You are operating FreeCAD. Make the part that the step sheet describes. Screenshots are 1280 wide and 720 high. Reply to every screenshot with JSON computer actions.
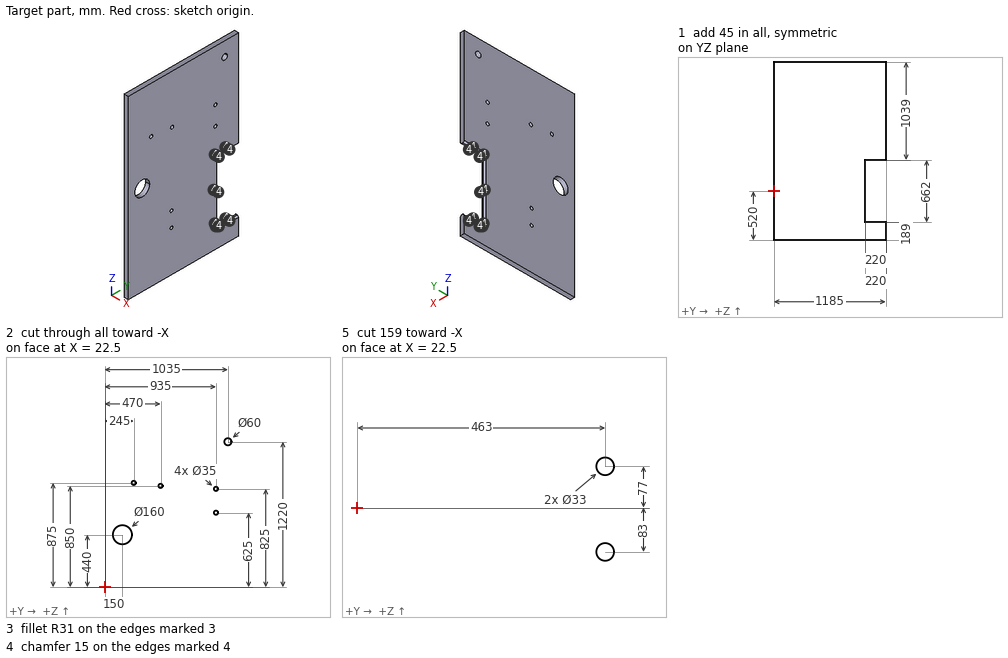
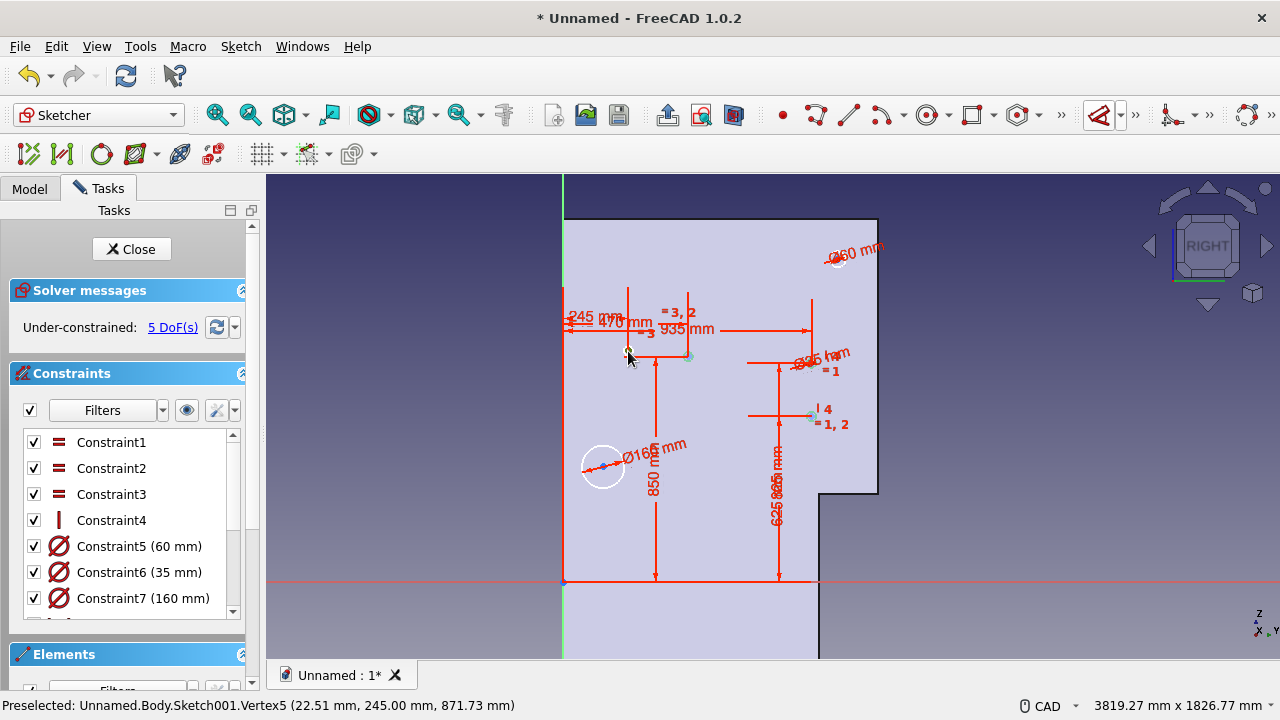
{"action": "left_click", "coordinate": [1120, 116]}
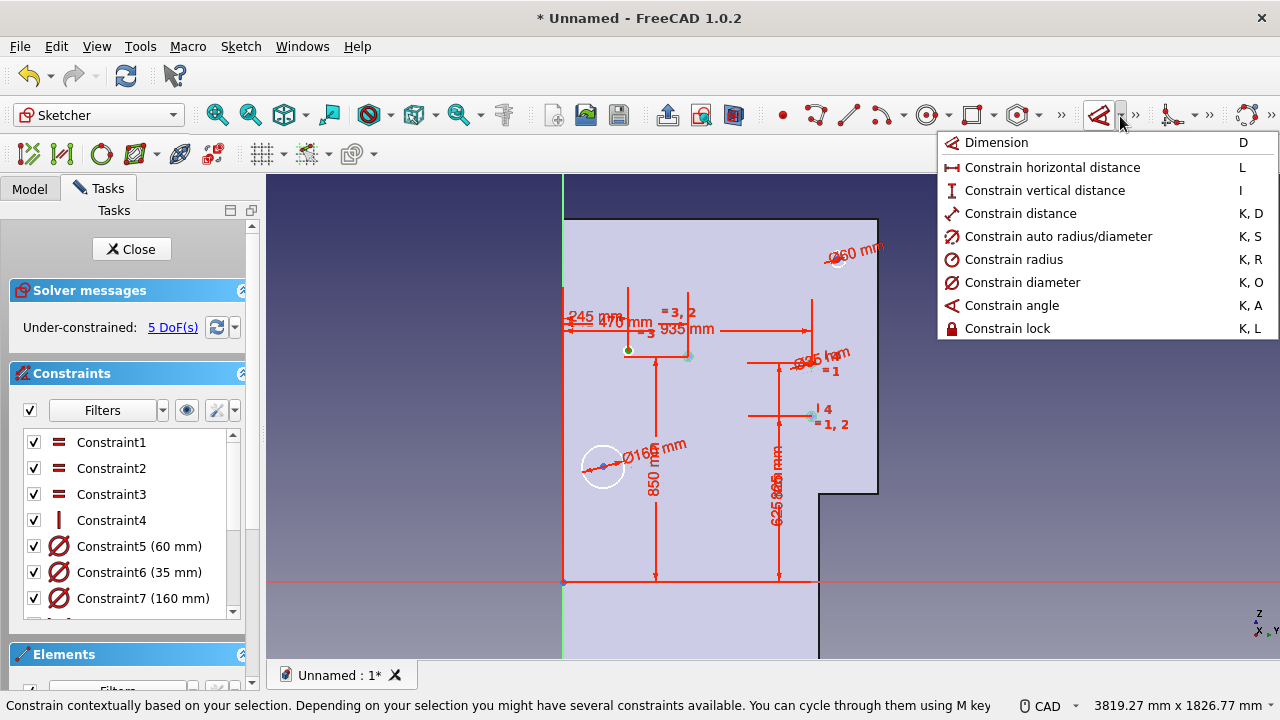
{"action": "left_click", "coordinate": [1108, 190]}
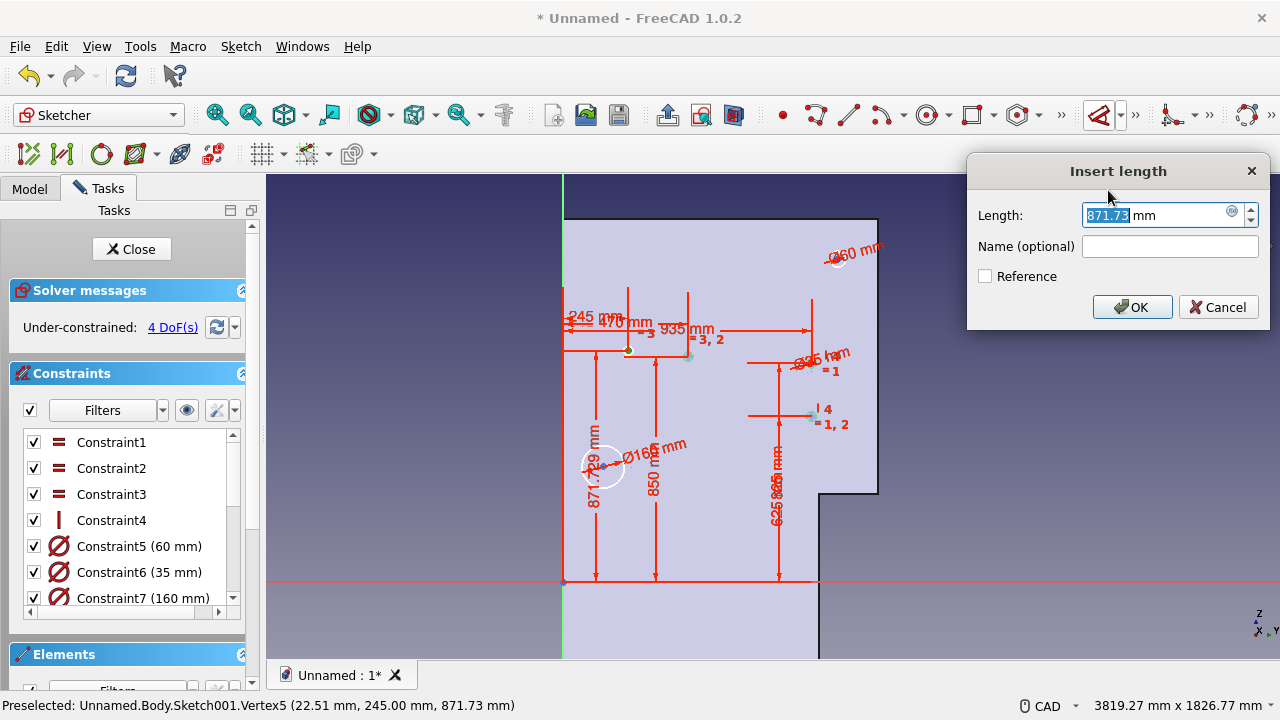
{"action": "type", "text": "875"}
{"action": "key", "text": "Return"}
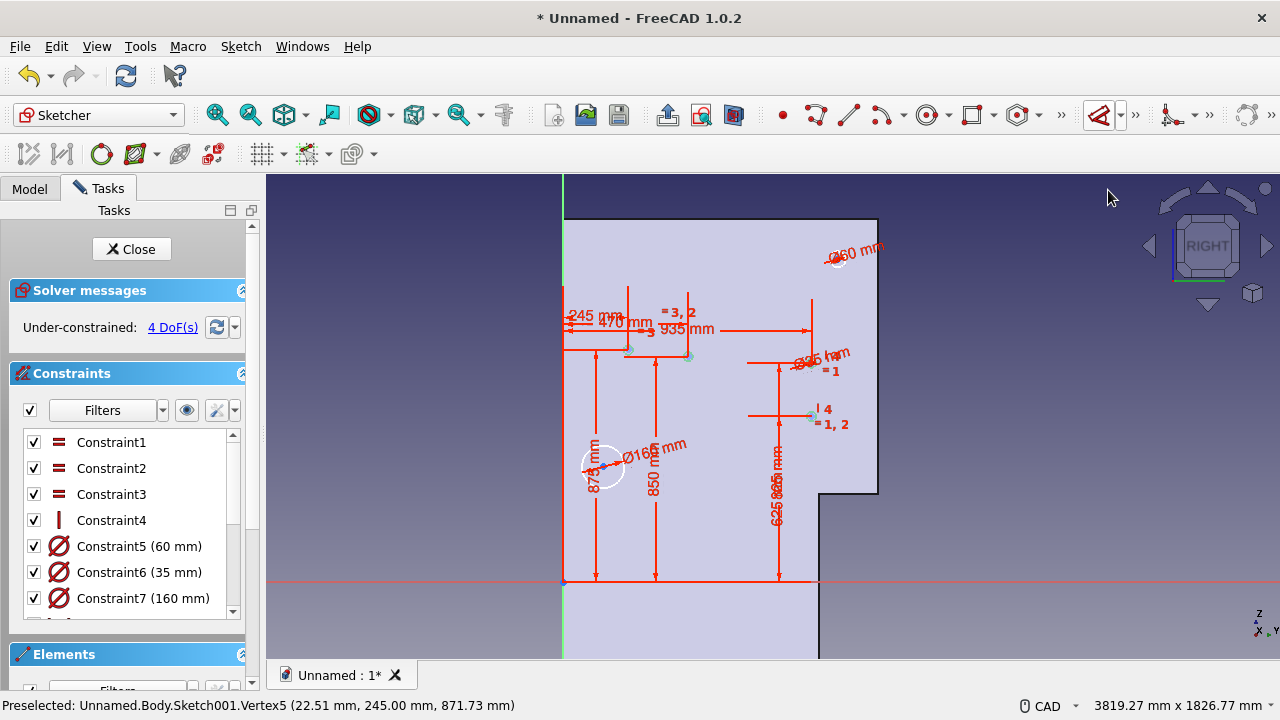
{"action": "left_click", "coordinate": [603, 467]}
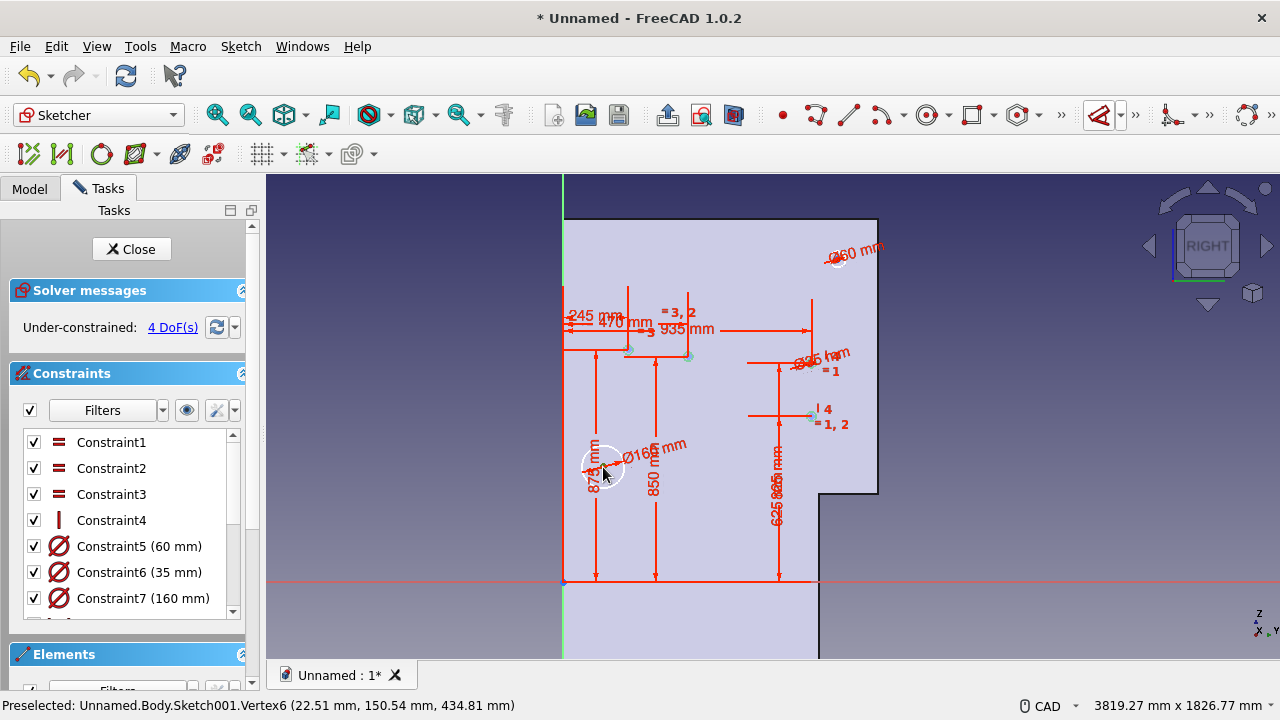
{"action": "left_click", "coordinate": [1120, 116]}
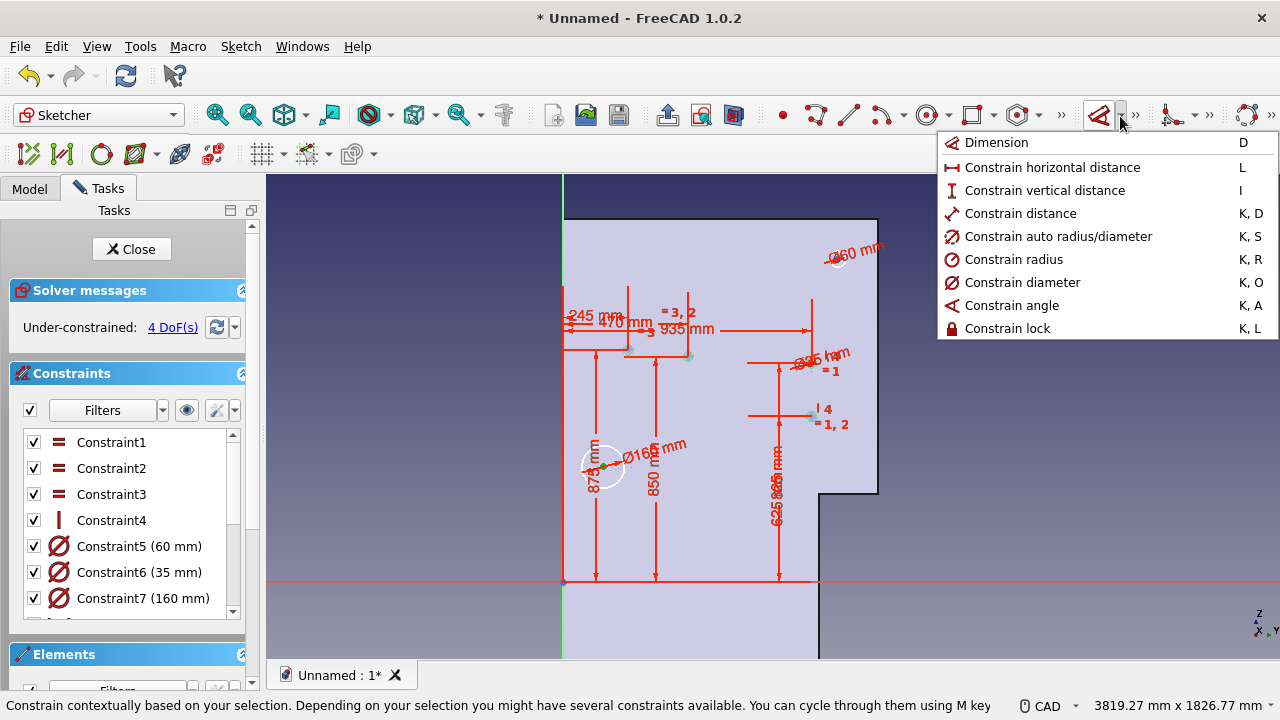
{"action": "left_click", "coordinate": [1108, 168]}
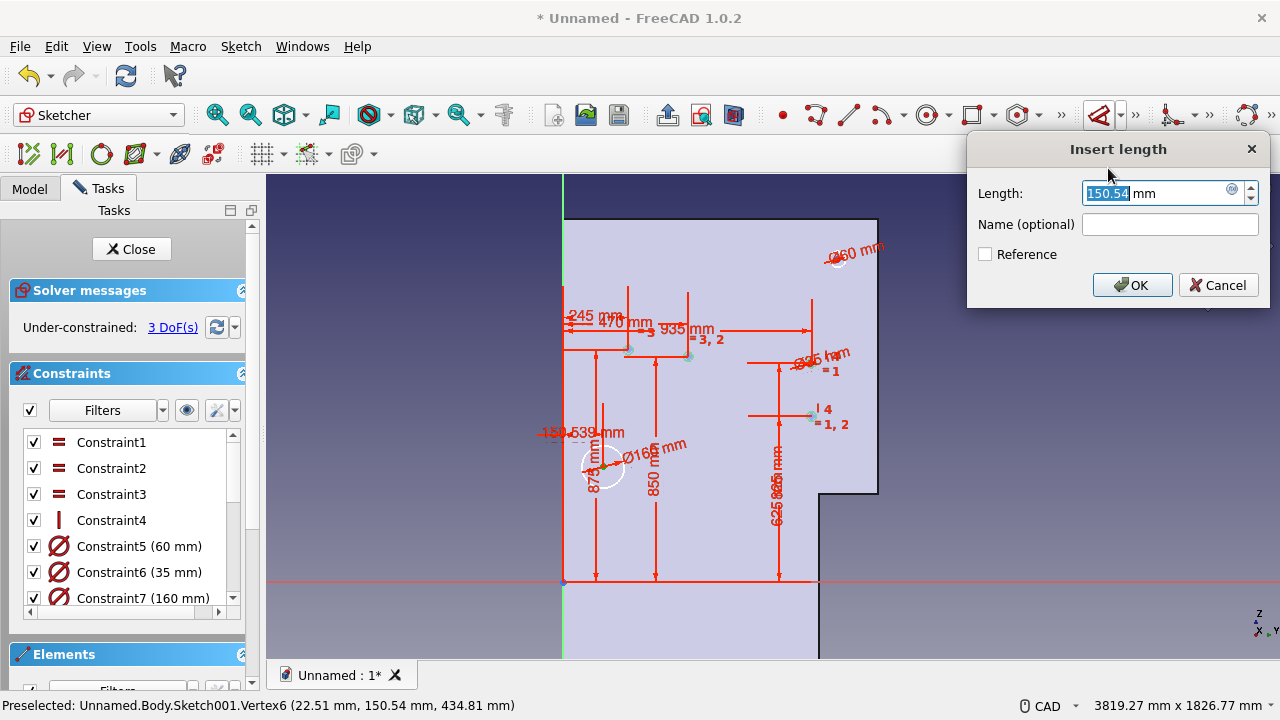
{"action": "type", "text": "150"}
{"action": "key", "text": "Return"}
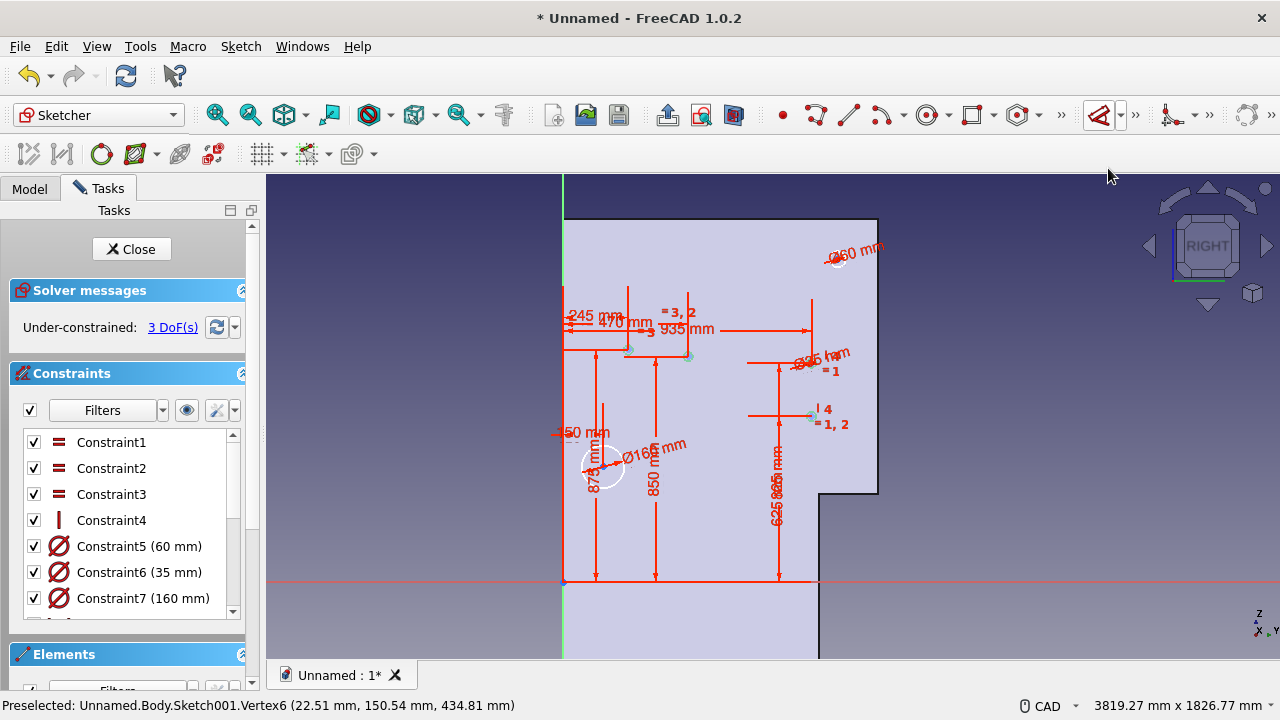
{"action": "left_click", "coordinate": [603, 467]}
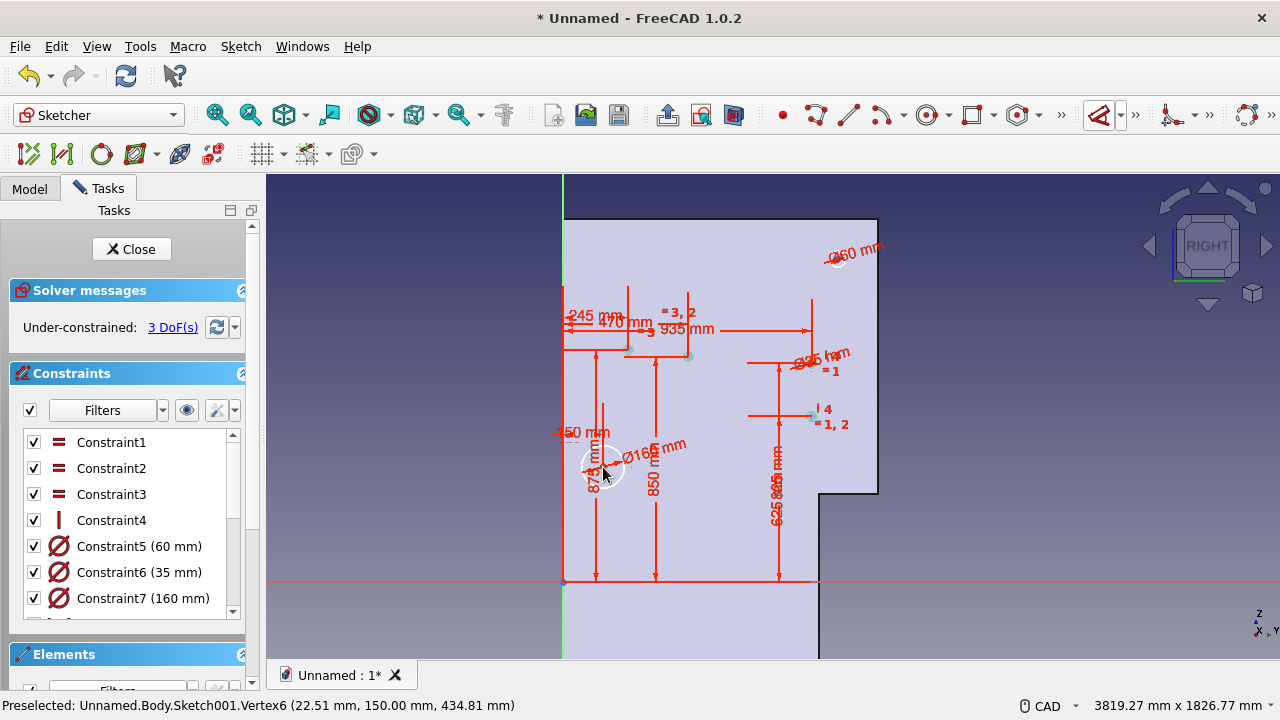
{"action": "left_click", "coordinate": [1120, 116]}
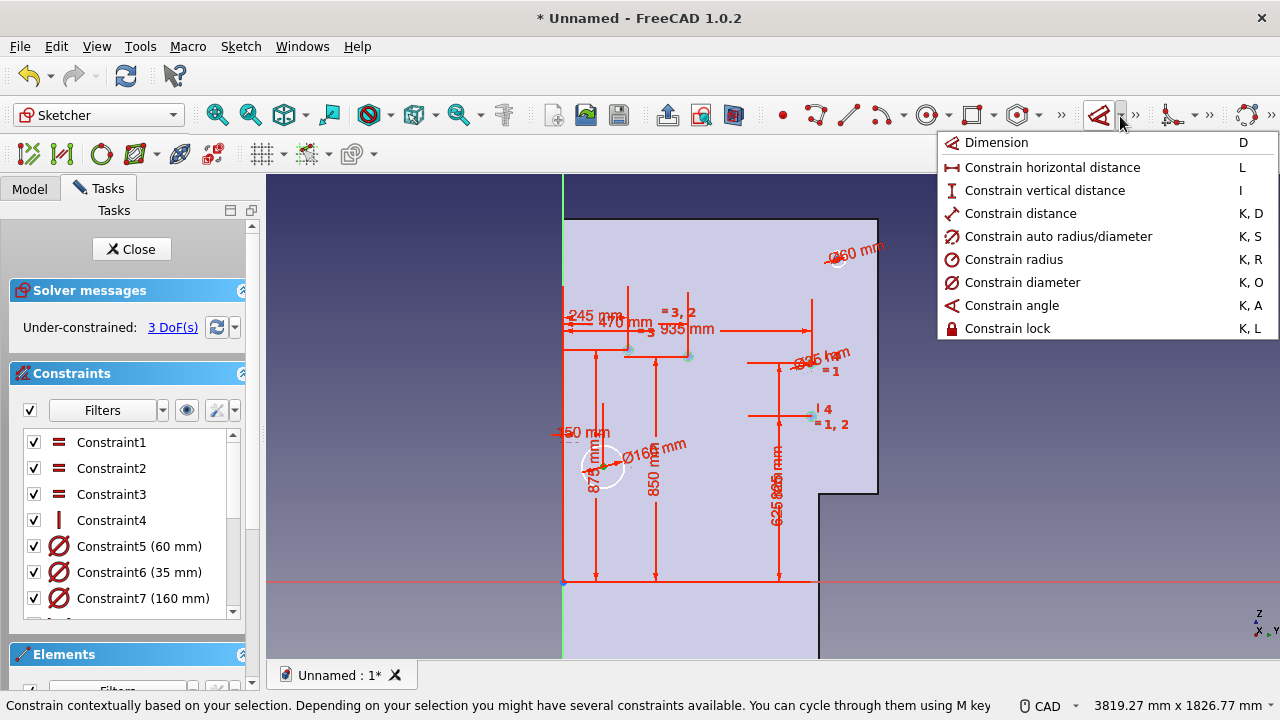
{"action": "left_click", "coordinate": [1108, 190]}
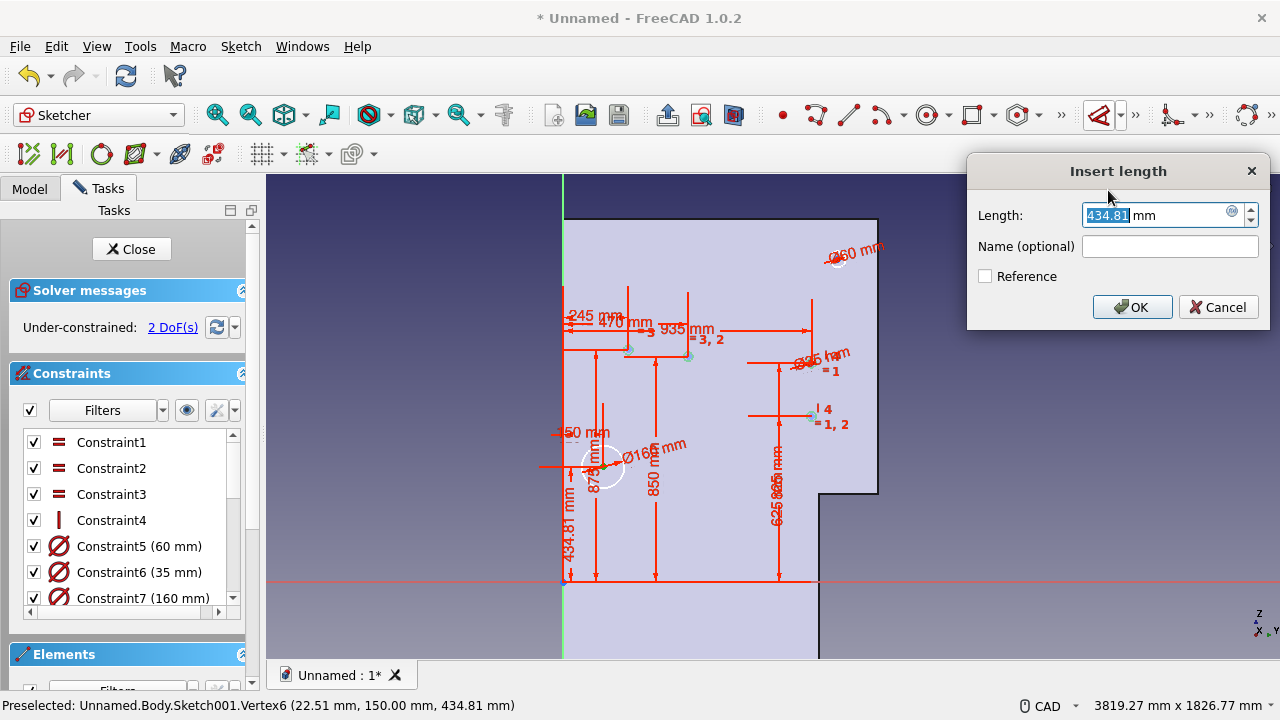
{"action": "type", "text": "440"}
{"action": "key", "text": "Return"}